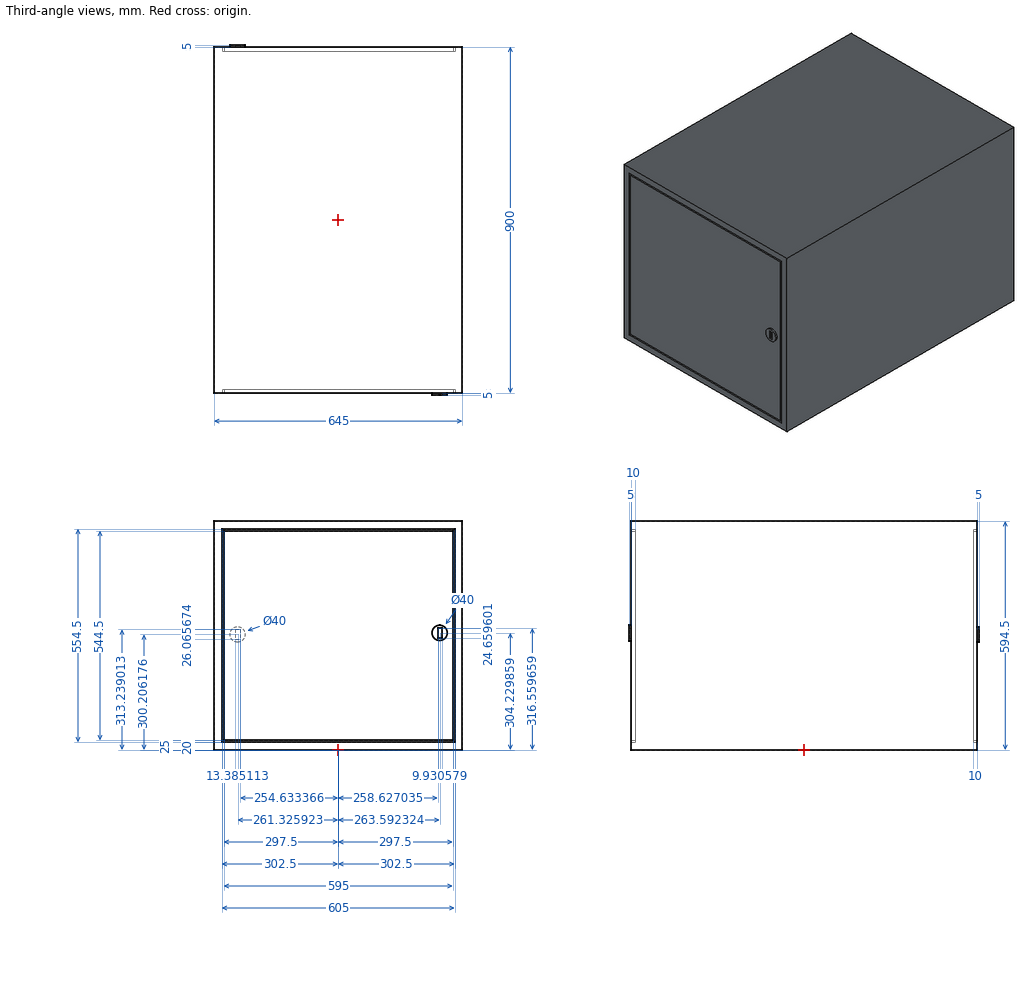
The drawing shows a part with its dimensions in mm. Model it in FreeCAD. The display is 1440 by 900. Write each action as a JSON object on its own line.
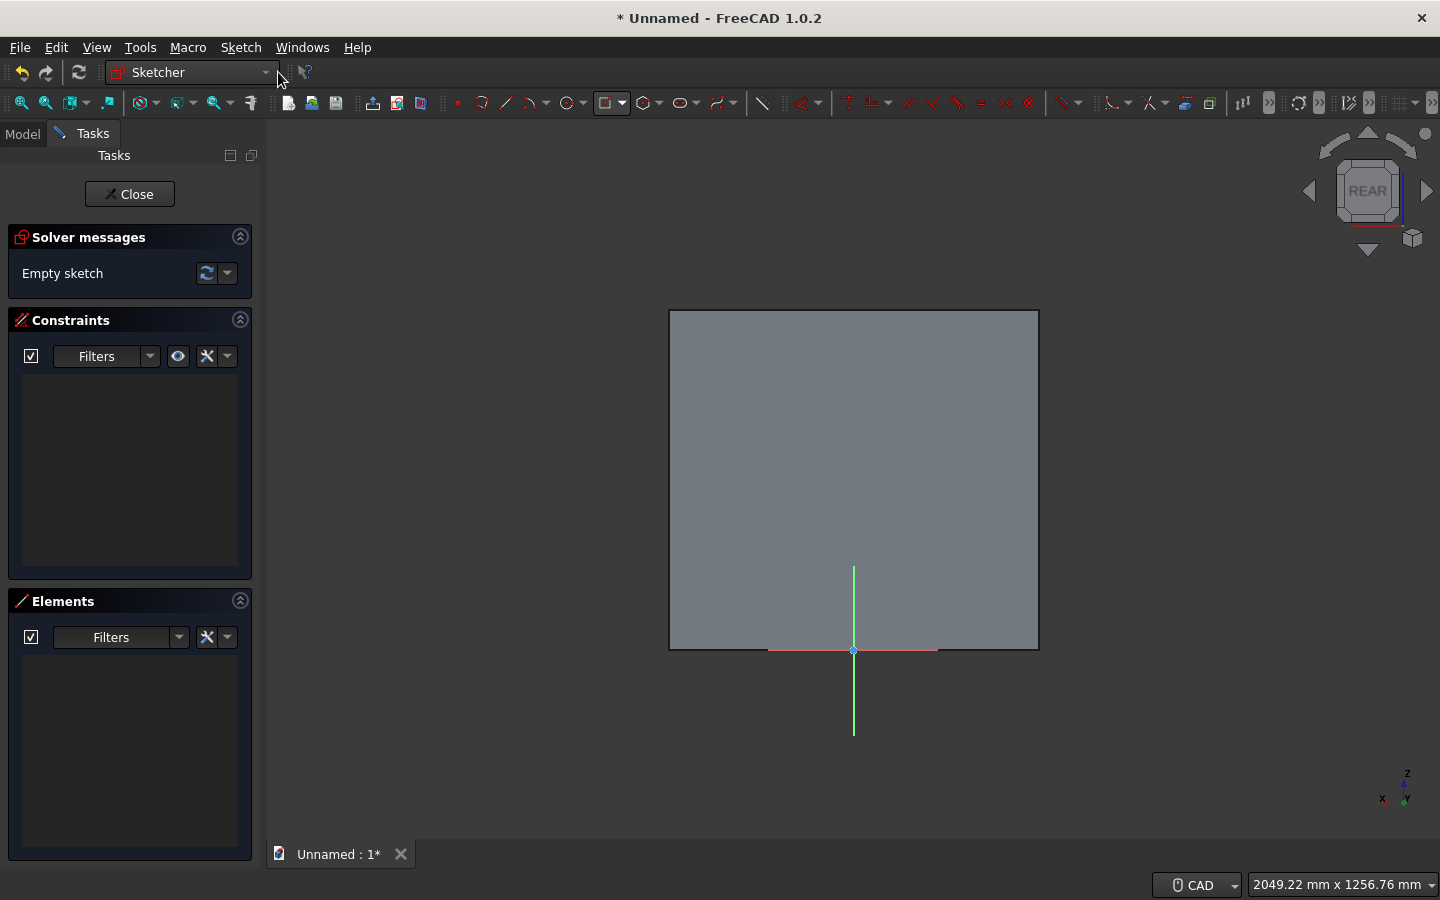
{"action": "scroll", "coordinate": [995, 500], "scroll_direction": "up", "scroll_amount": 2}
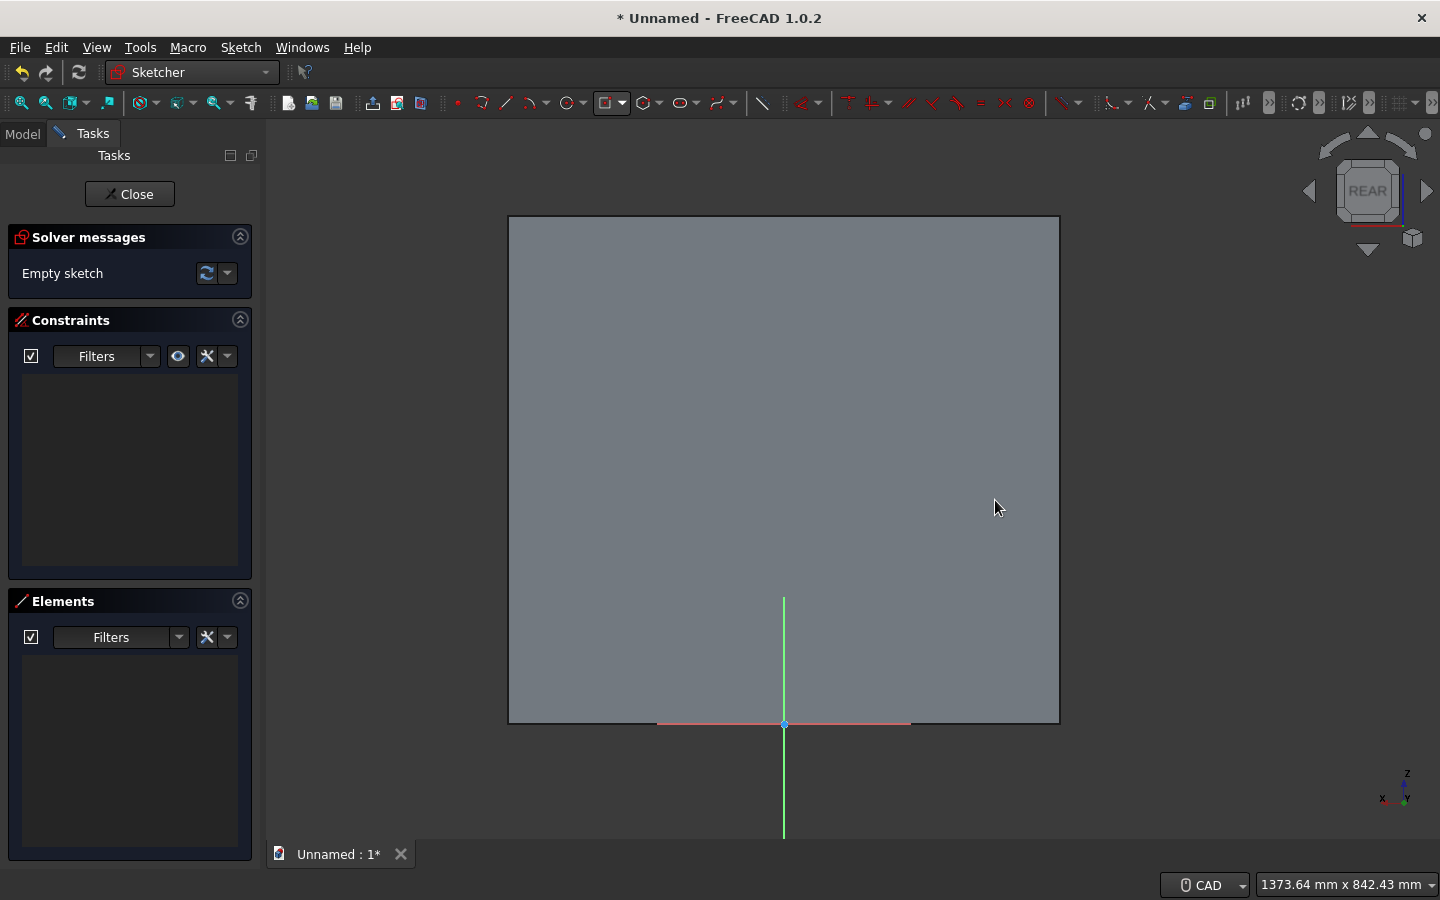
{"action": "key", "text": "g r"}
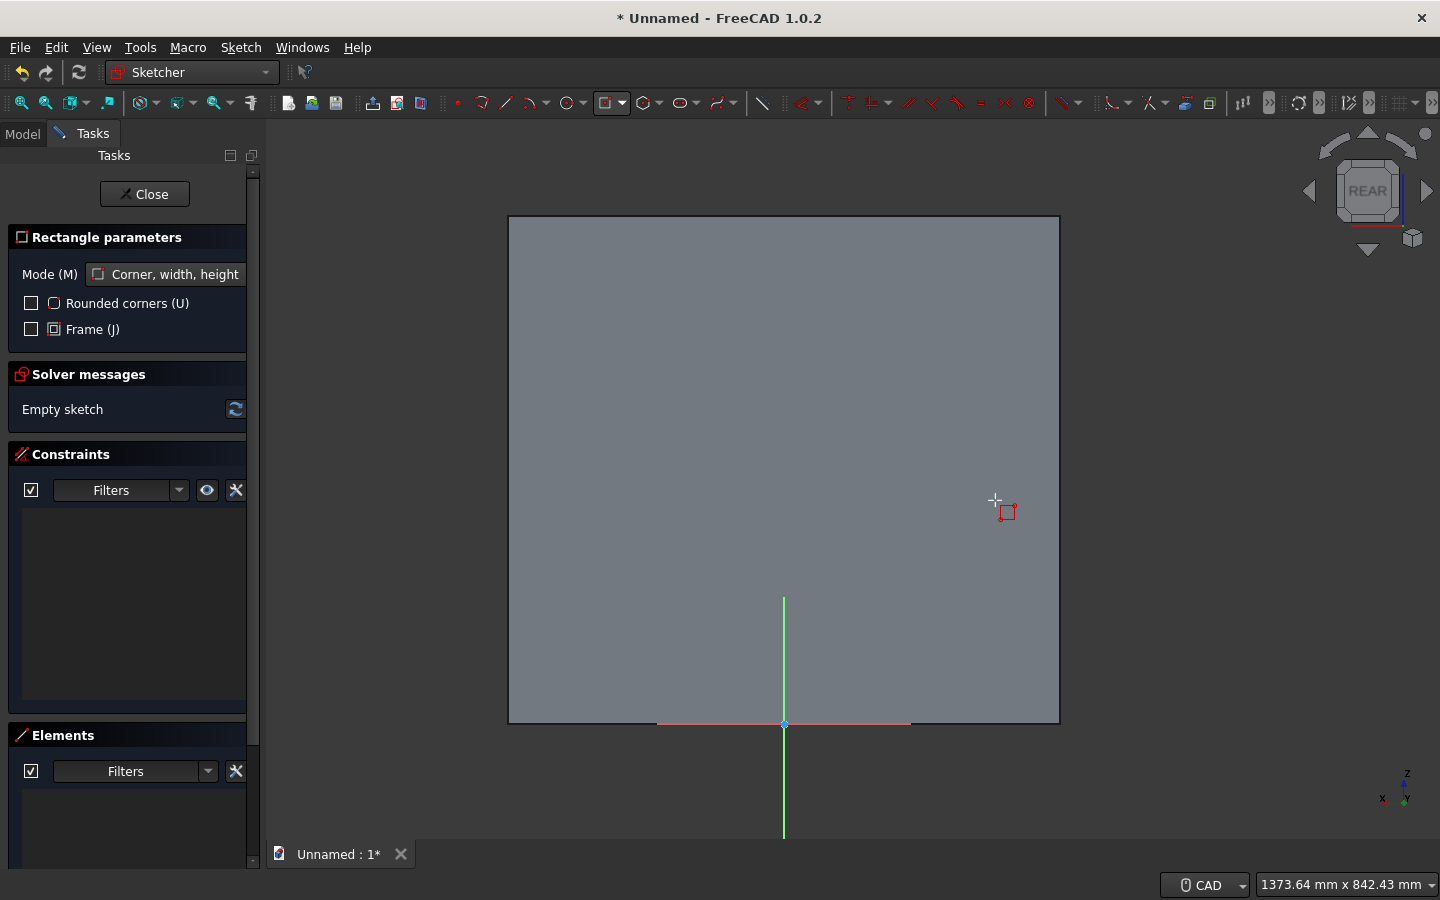
{"action": "left_click", "coordinate": [526, 233]}
{"action": "left_click", "coordinate": [1043, 707]}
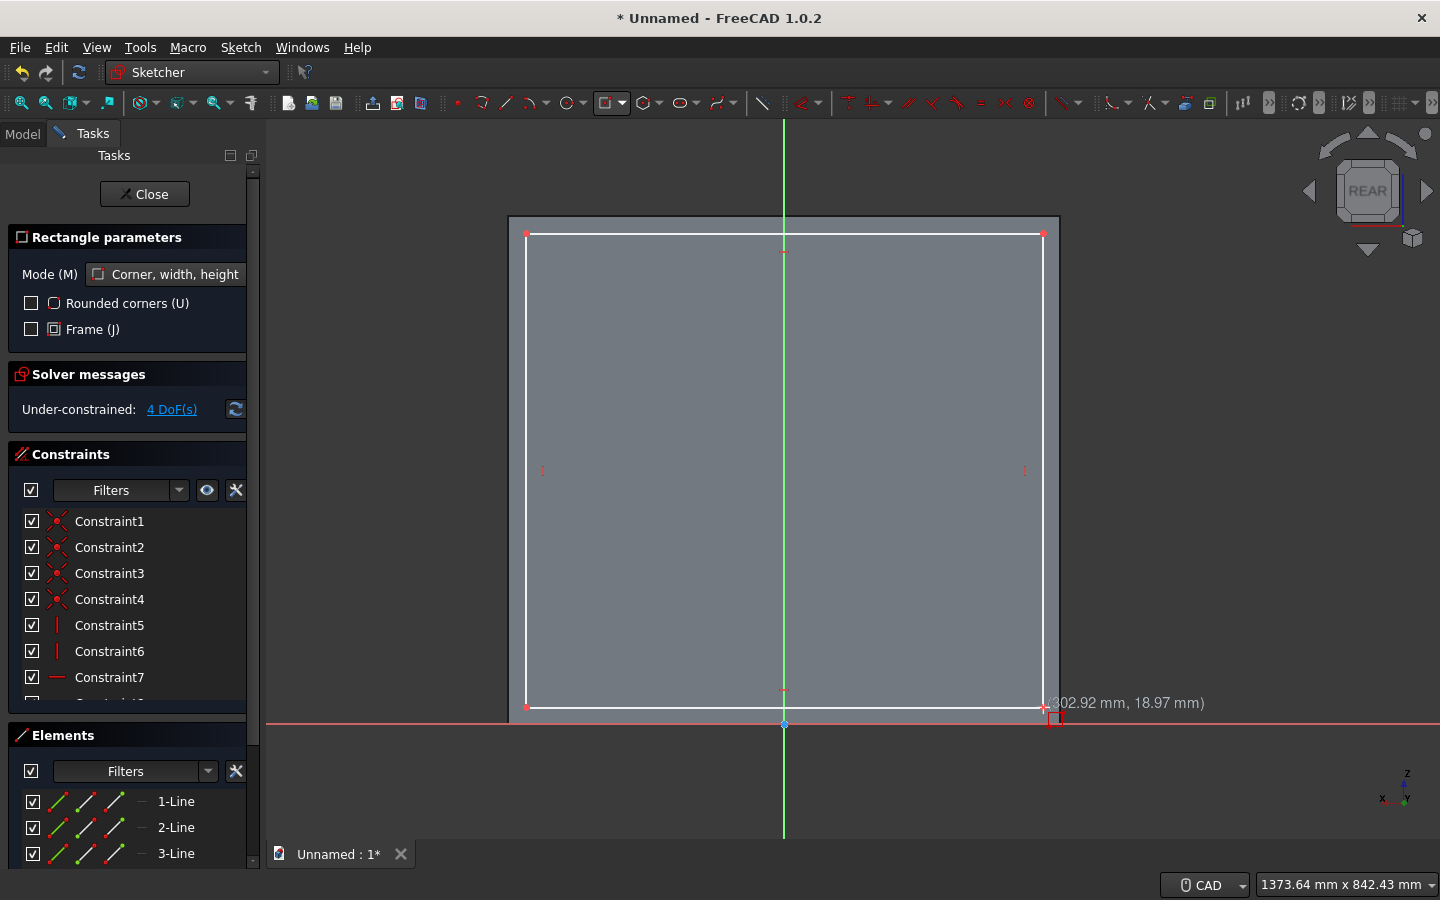
{"action": "scroll", "coordinate": [530, 237], "scroll_direction": "up", "scroll_amount": 7}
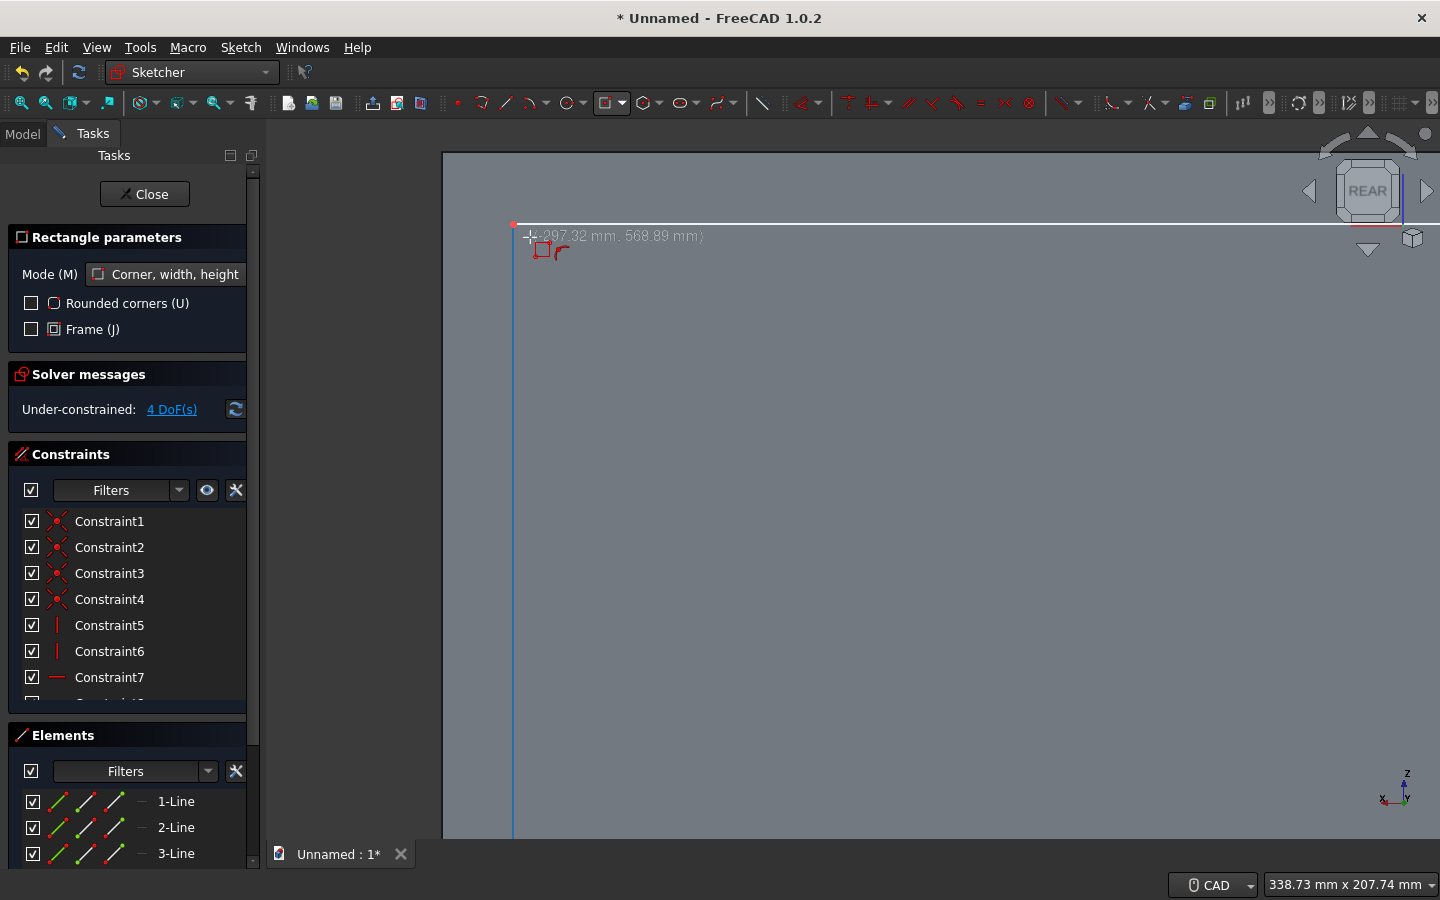
{"action": "left_click", "coordinate": [529, 238]}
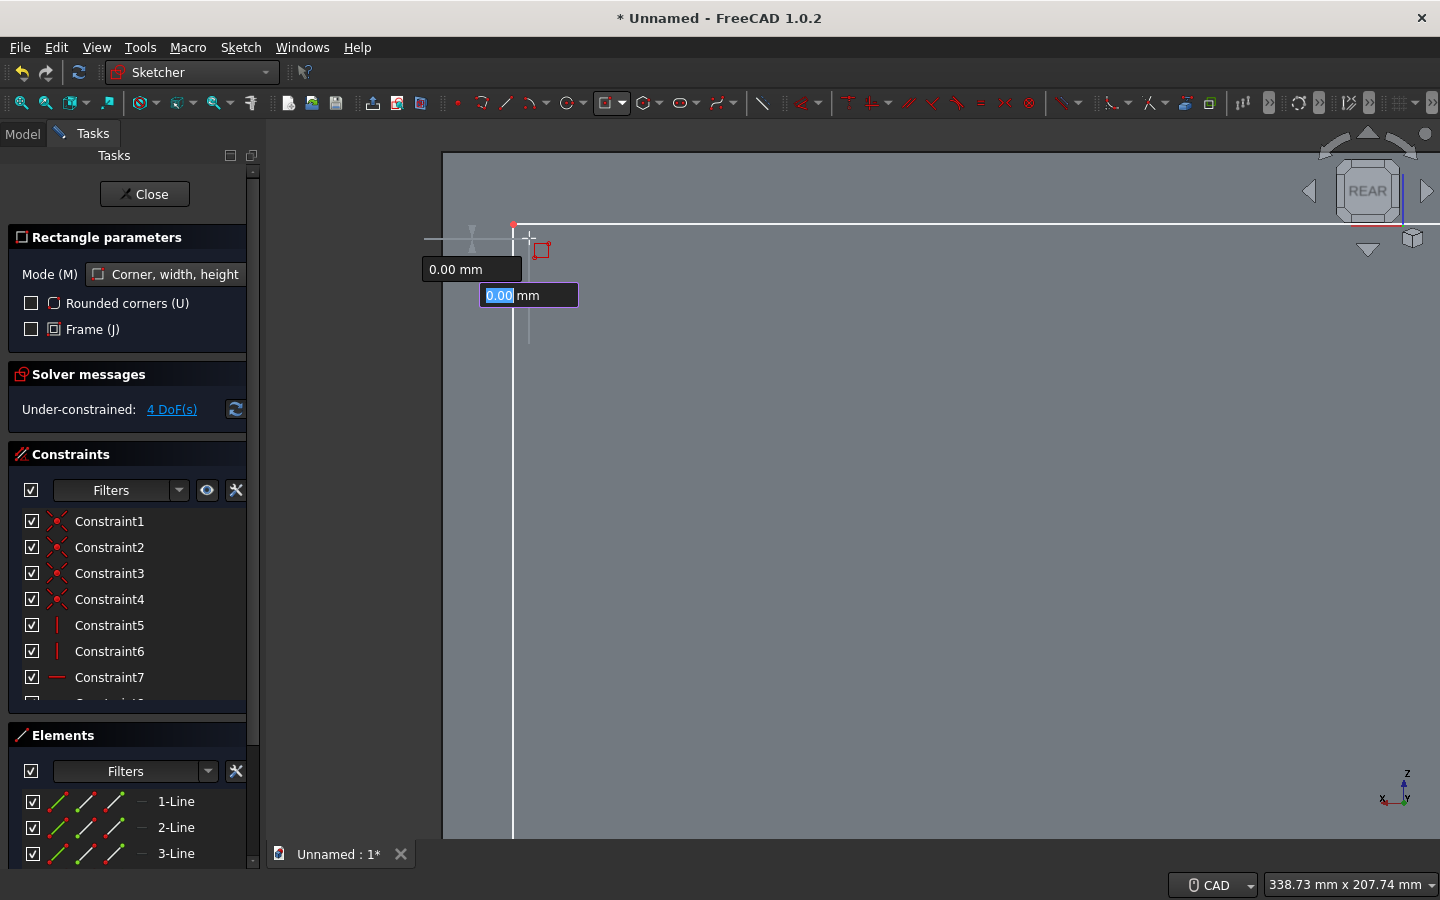
{"action": "scroll", "coordinate": [531, 238], "scroll_direction": "down", "scroll_amount": 7}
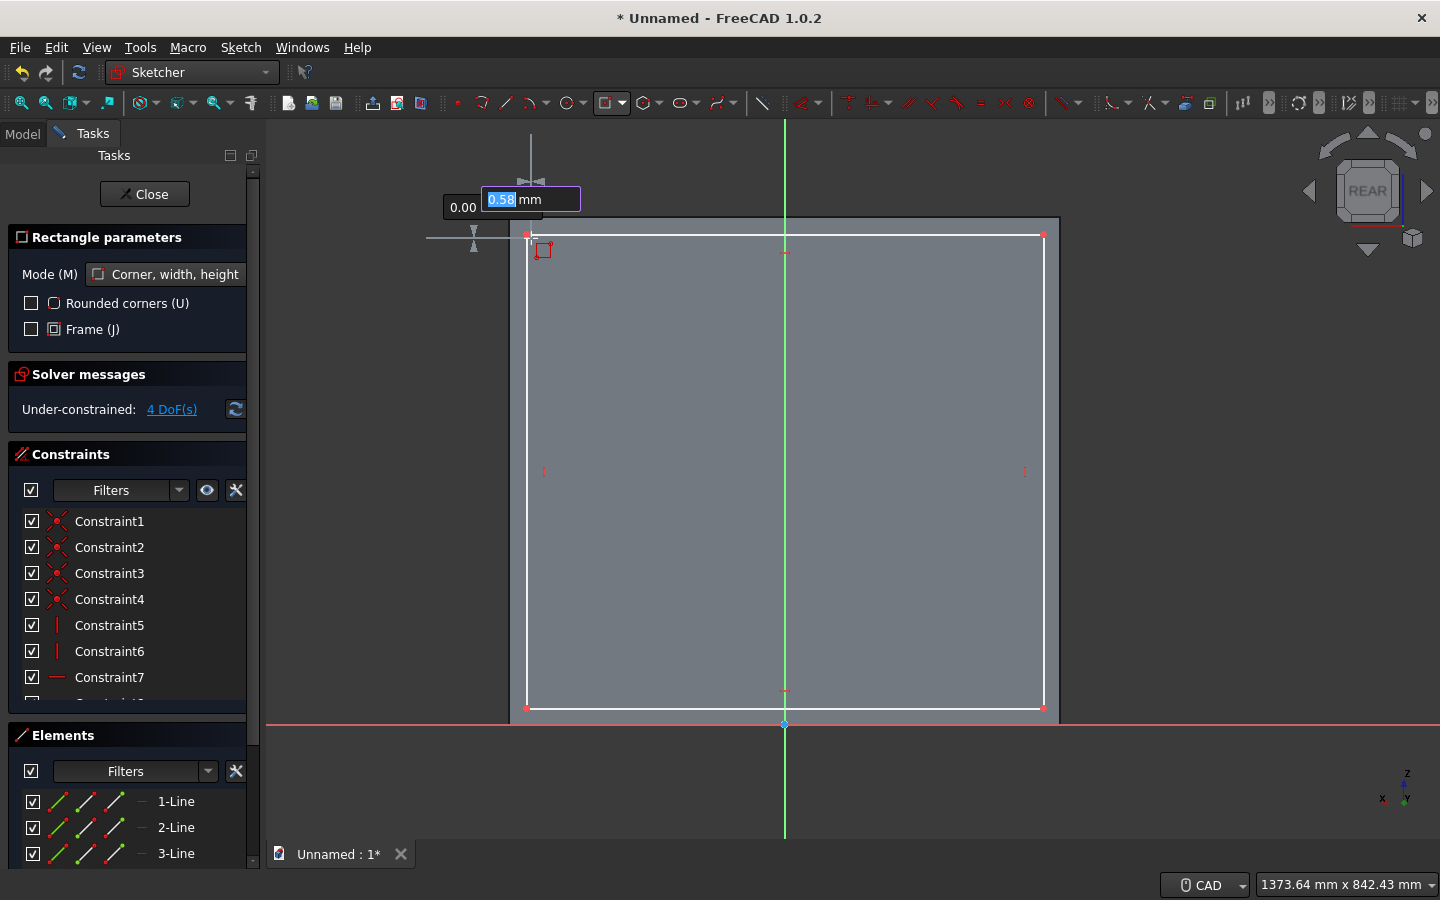
{"action": "scroll", "coordinate": [1039, 704], "scroll_direction": "up", "scroll_amount": 7}